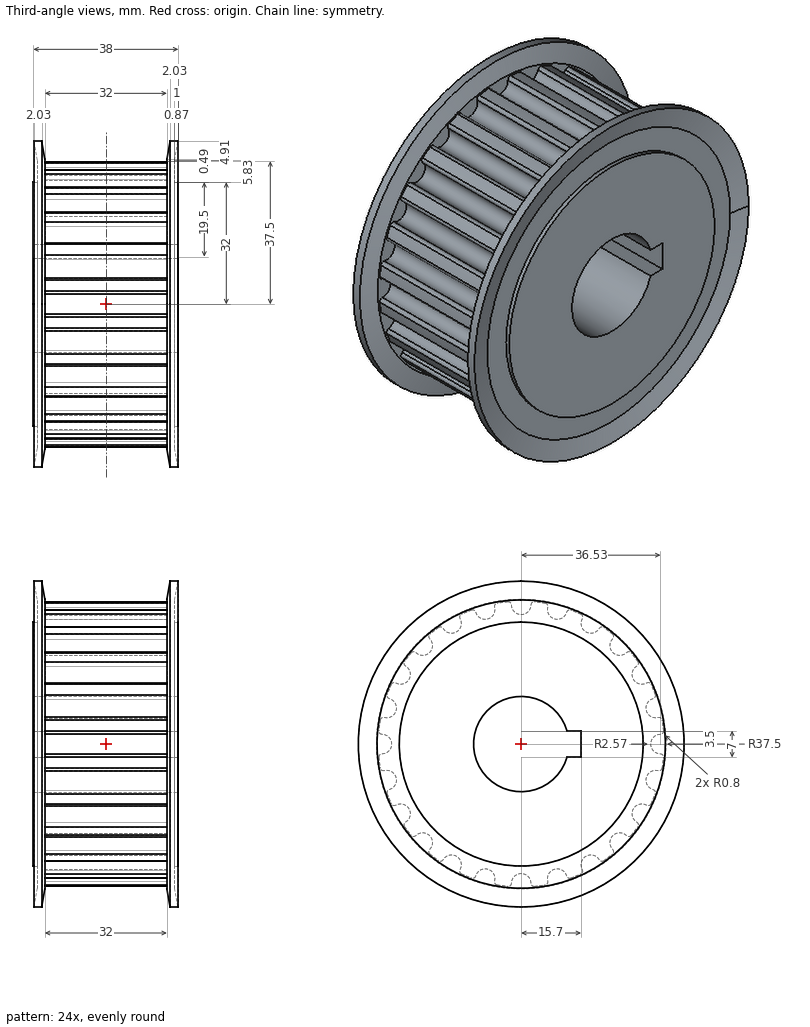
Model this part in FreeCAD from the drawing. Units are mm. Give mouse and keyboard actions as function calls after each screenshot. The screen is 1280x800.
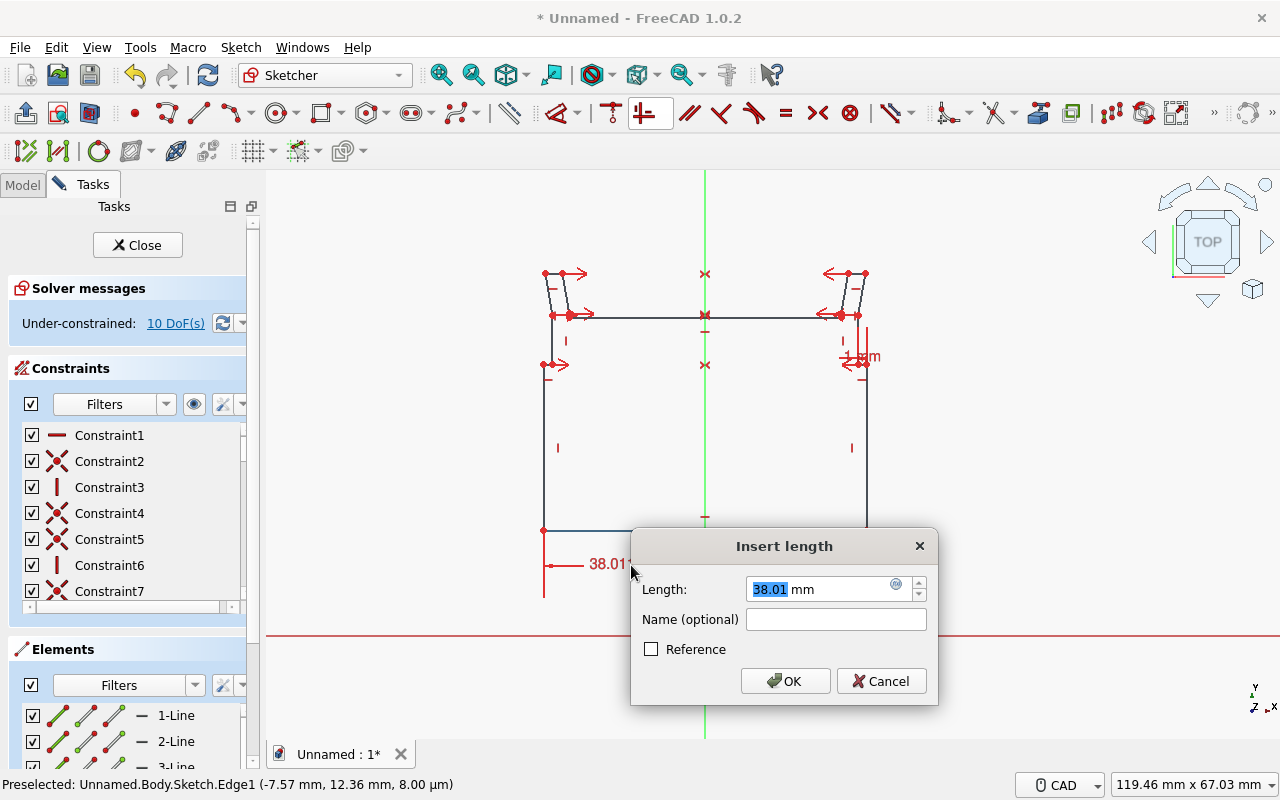
text(38)
key(Return)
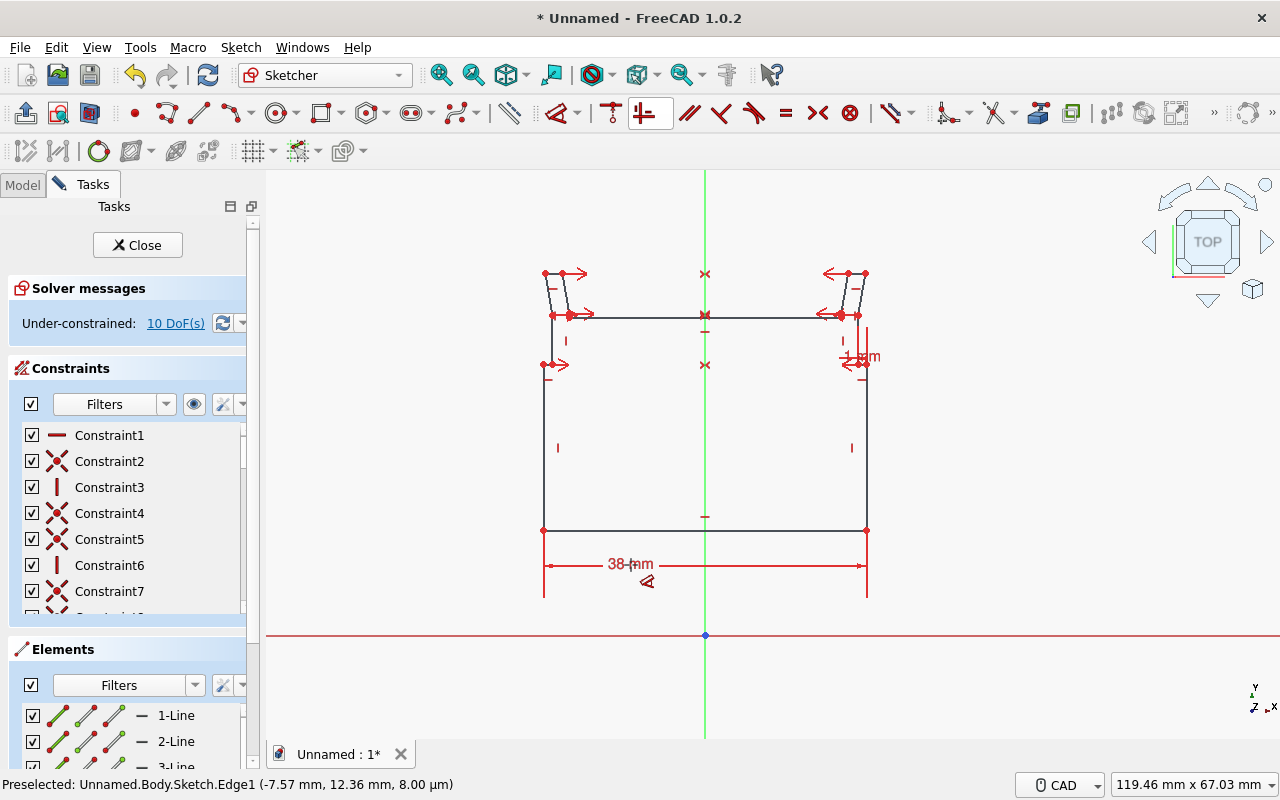
click(760, 318)
click(643, 284)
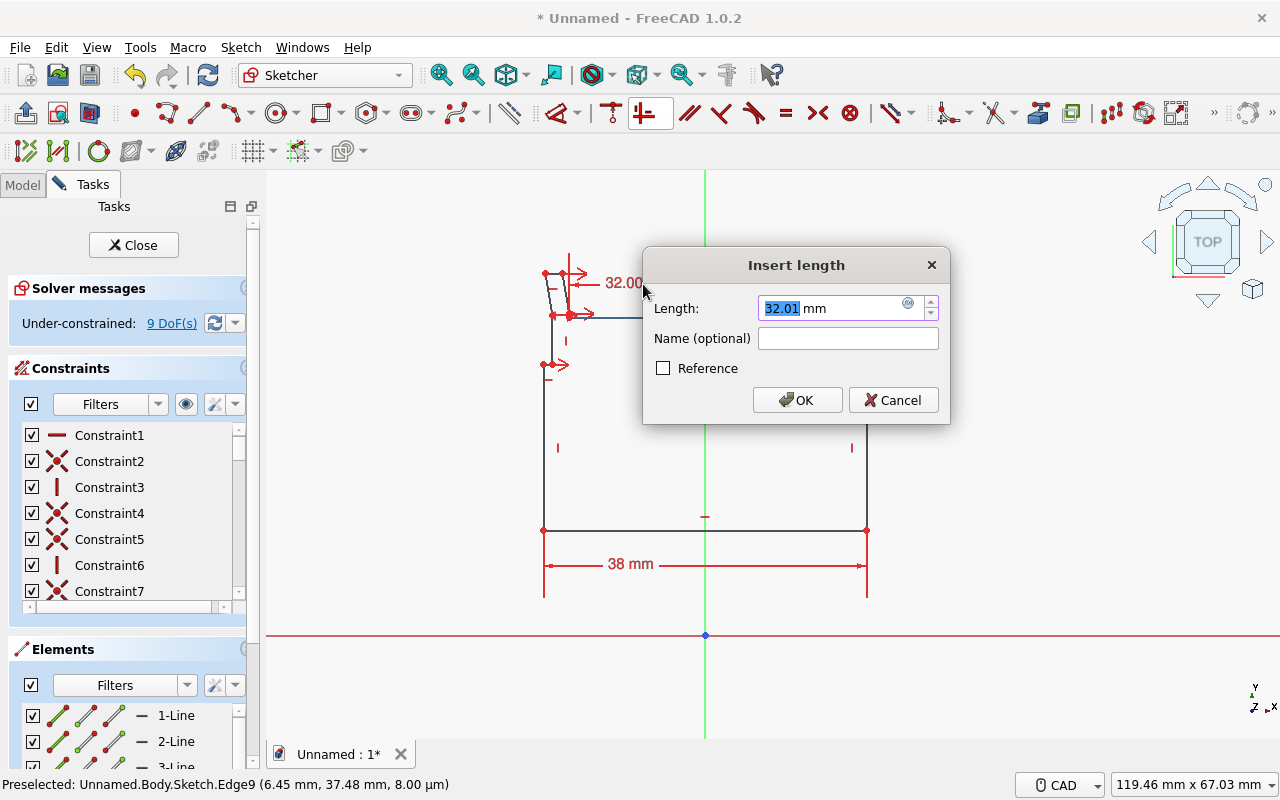
text(32)
key(Return)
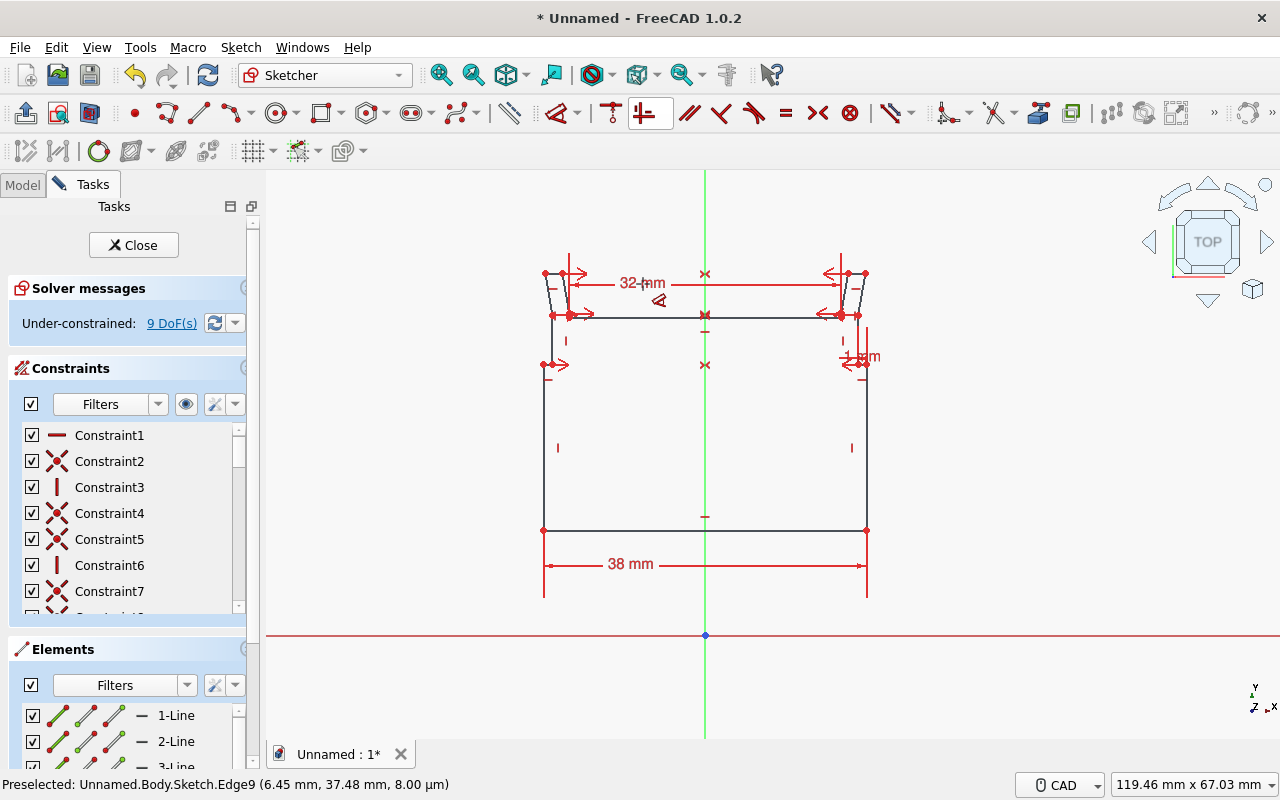
scroll(867, 365, up, 2)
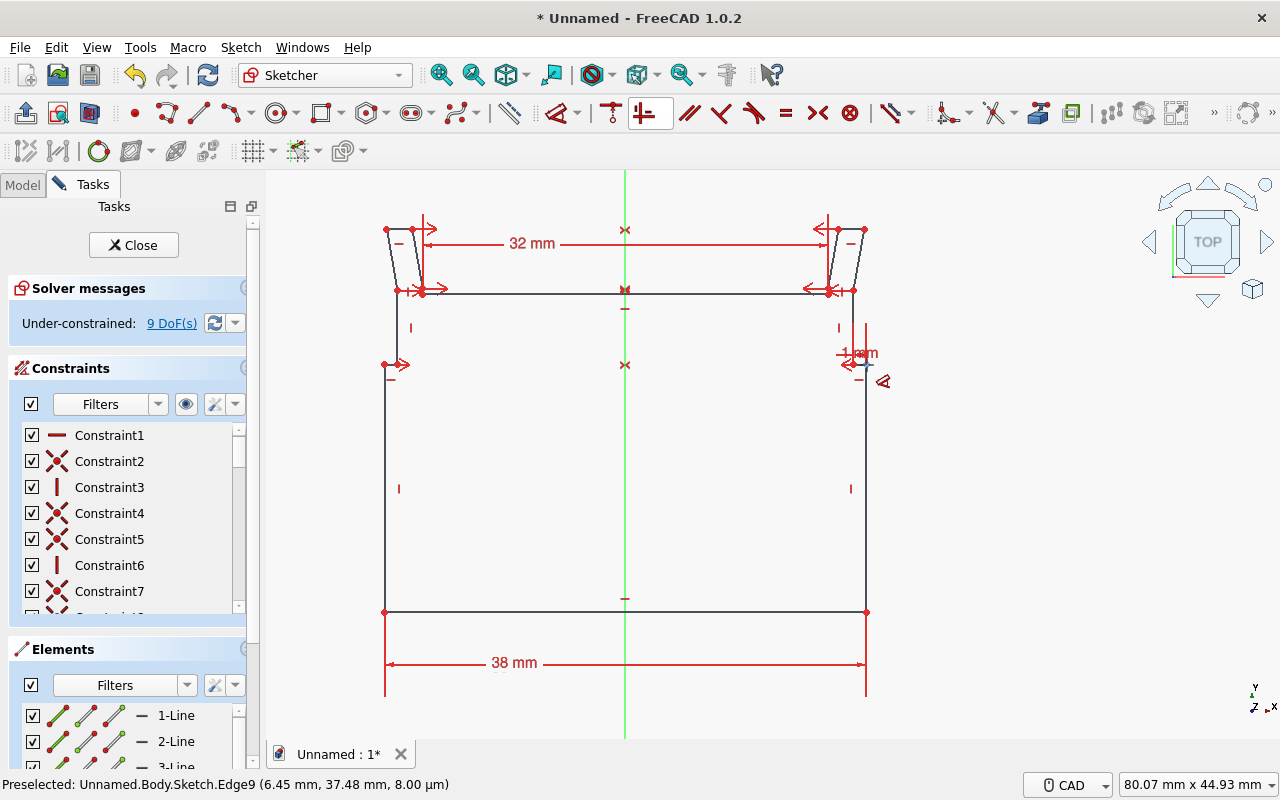
click(866, 365)
click(900, 538)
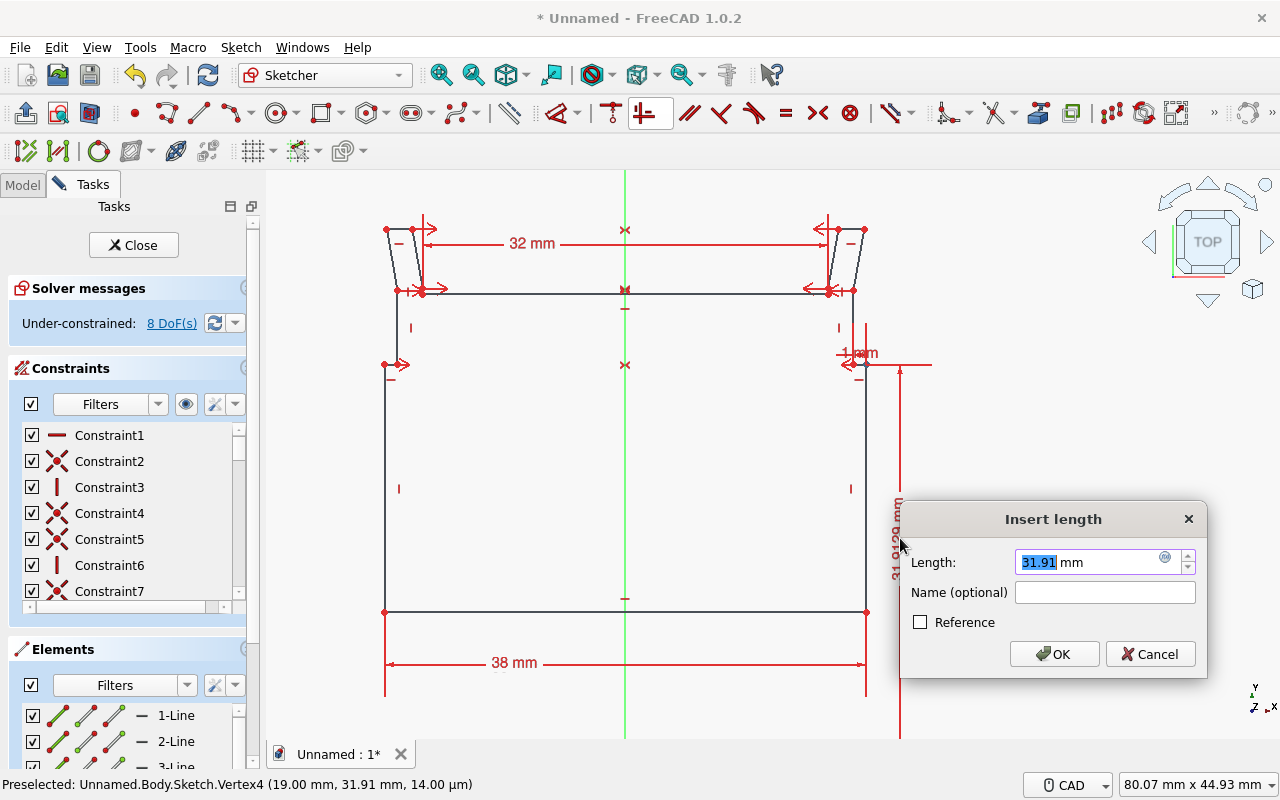
text(32)
key(Return)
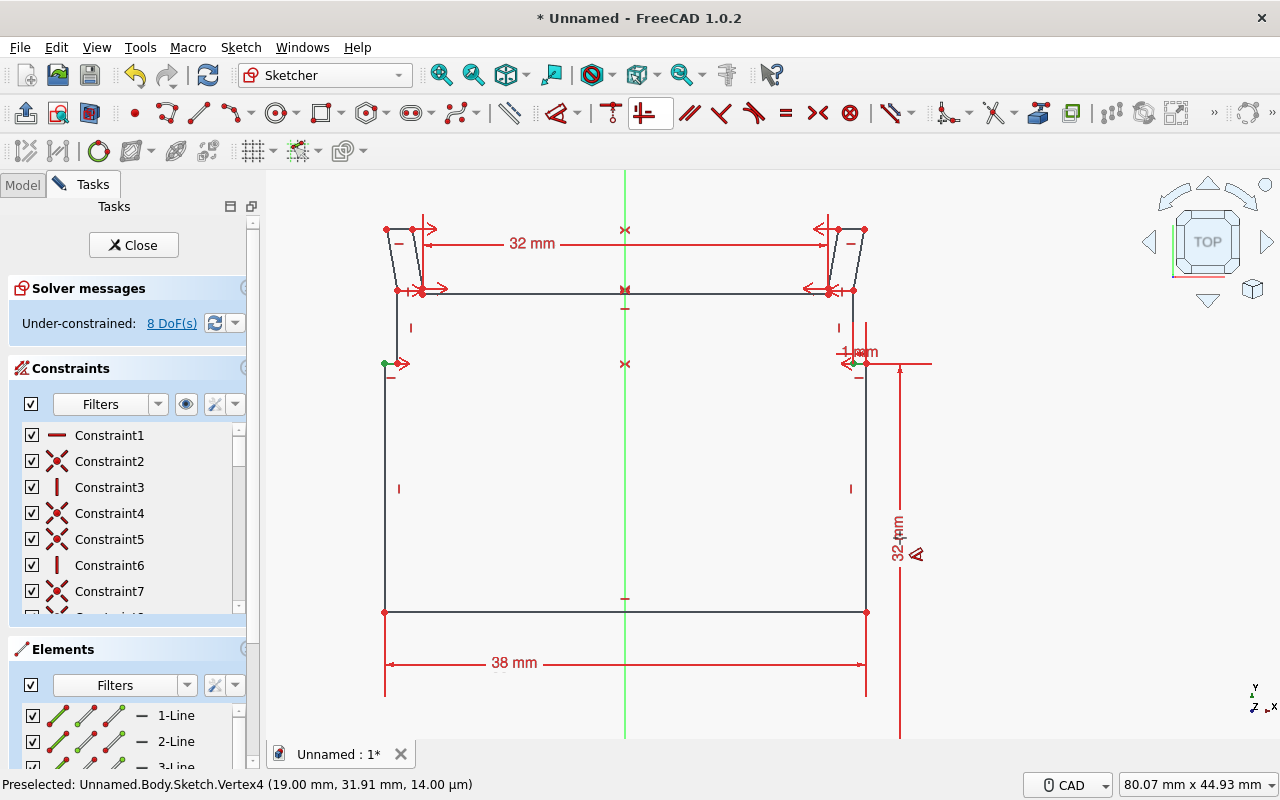
click(866, 538)
click(900, 488)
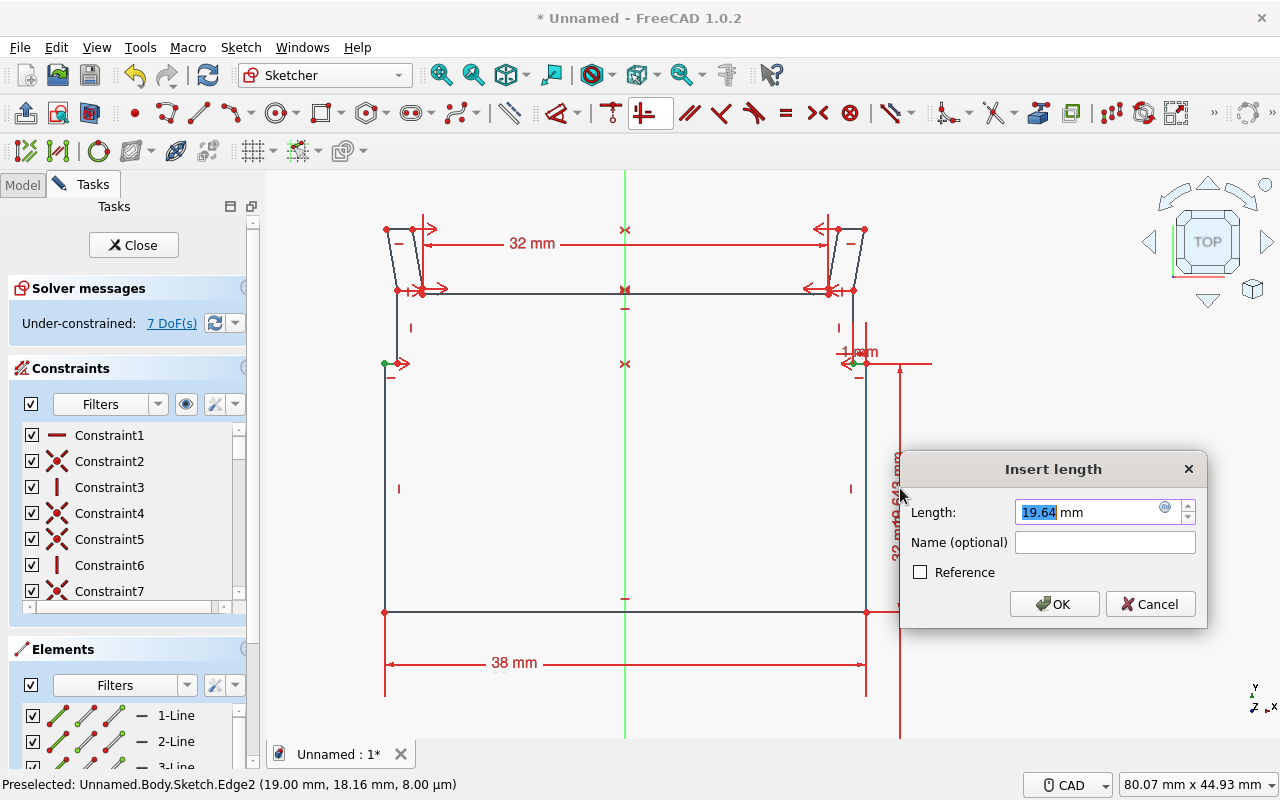
text(19.5)
key(Return)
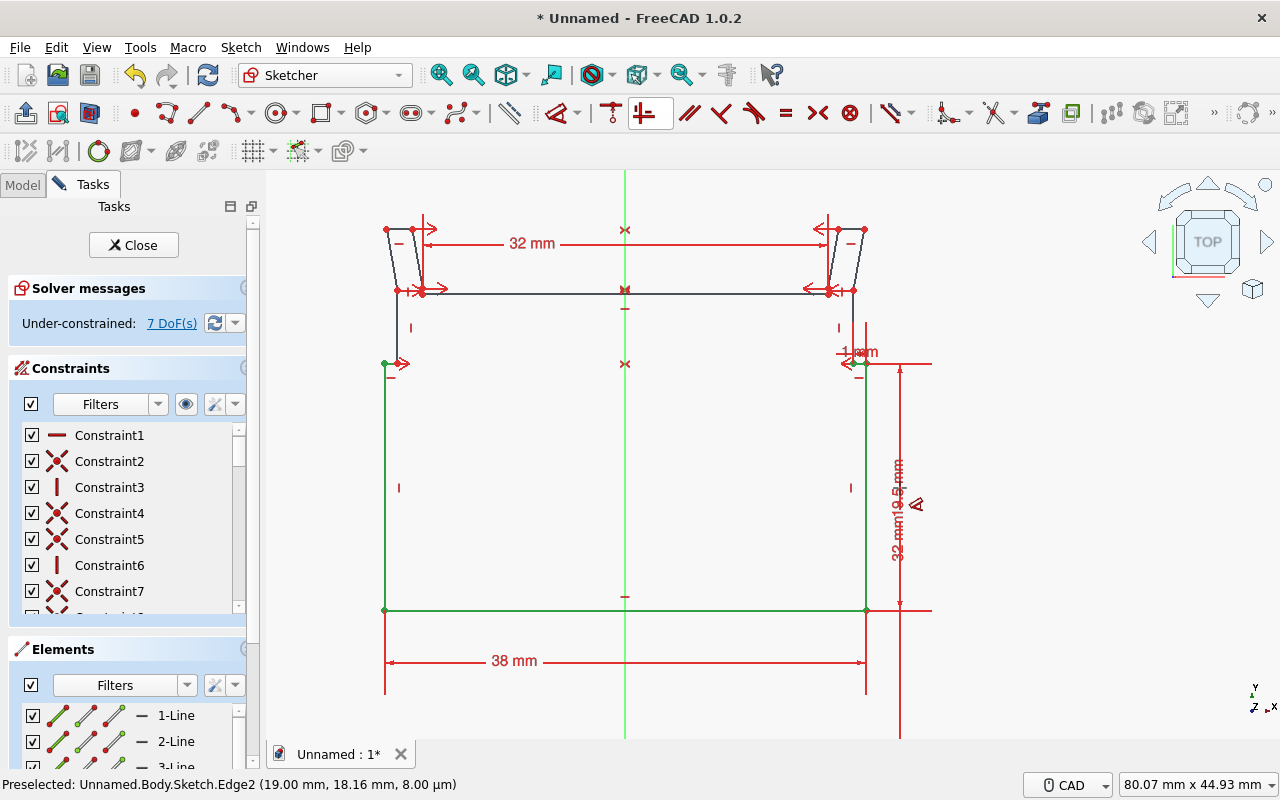
click(853, 342)
click(887, 327)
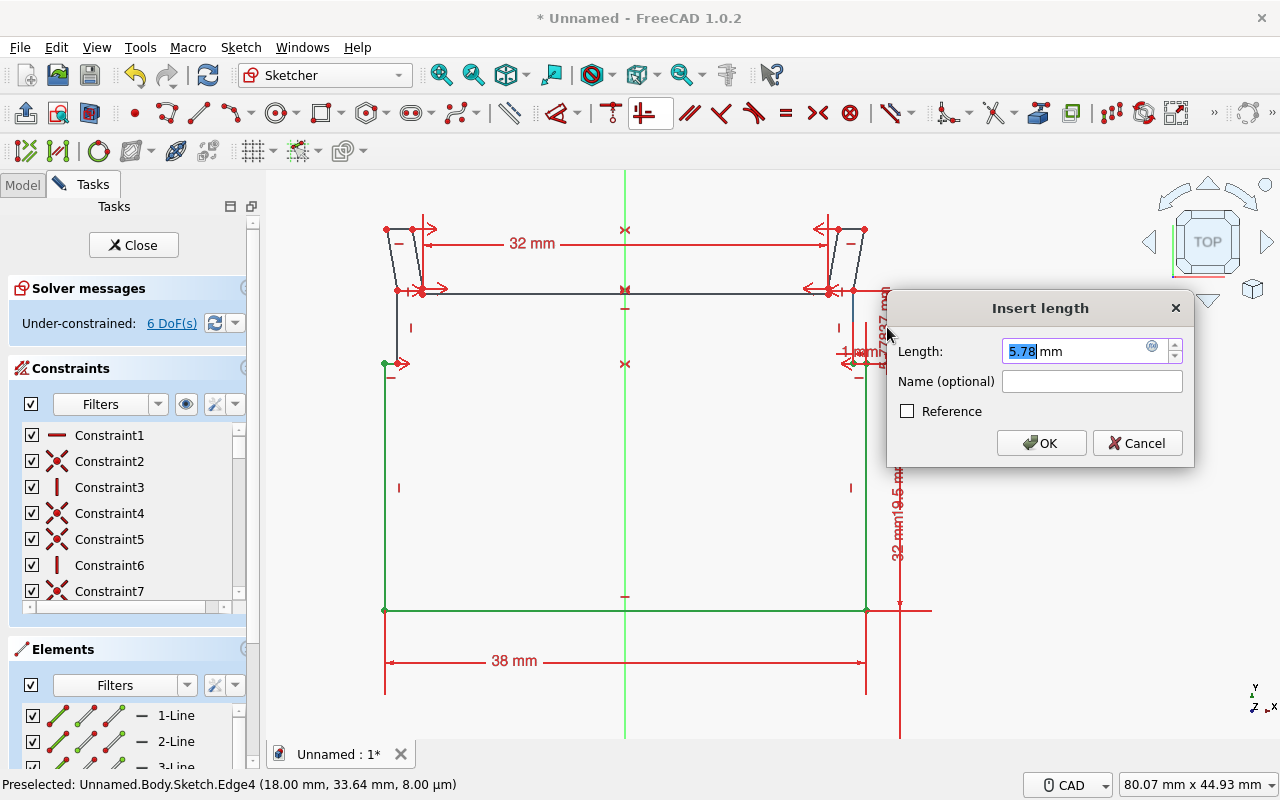
text(5.83)
key(Return)